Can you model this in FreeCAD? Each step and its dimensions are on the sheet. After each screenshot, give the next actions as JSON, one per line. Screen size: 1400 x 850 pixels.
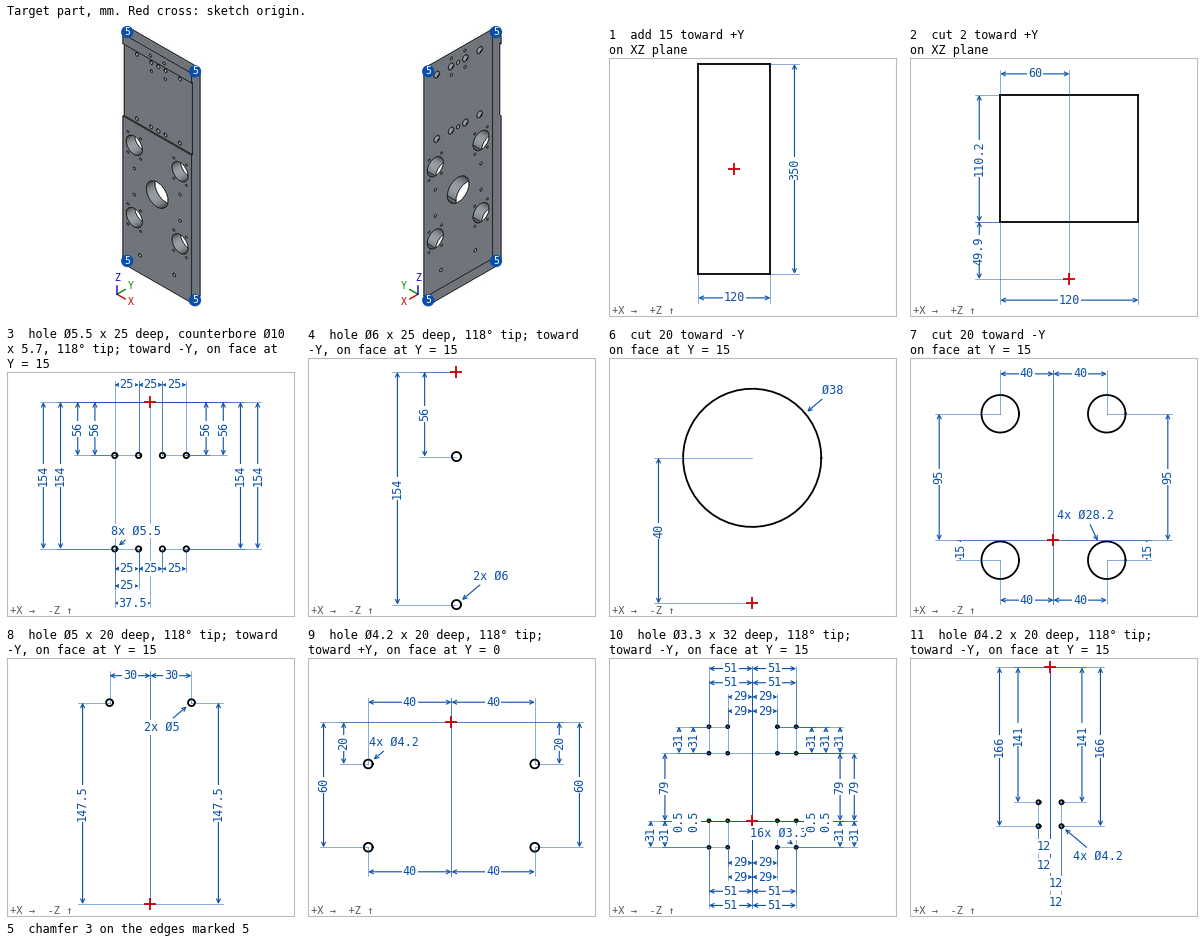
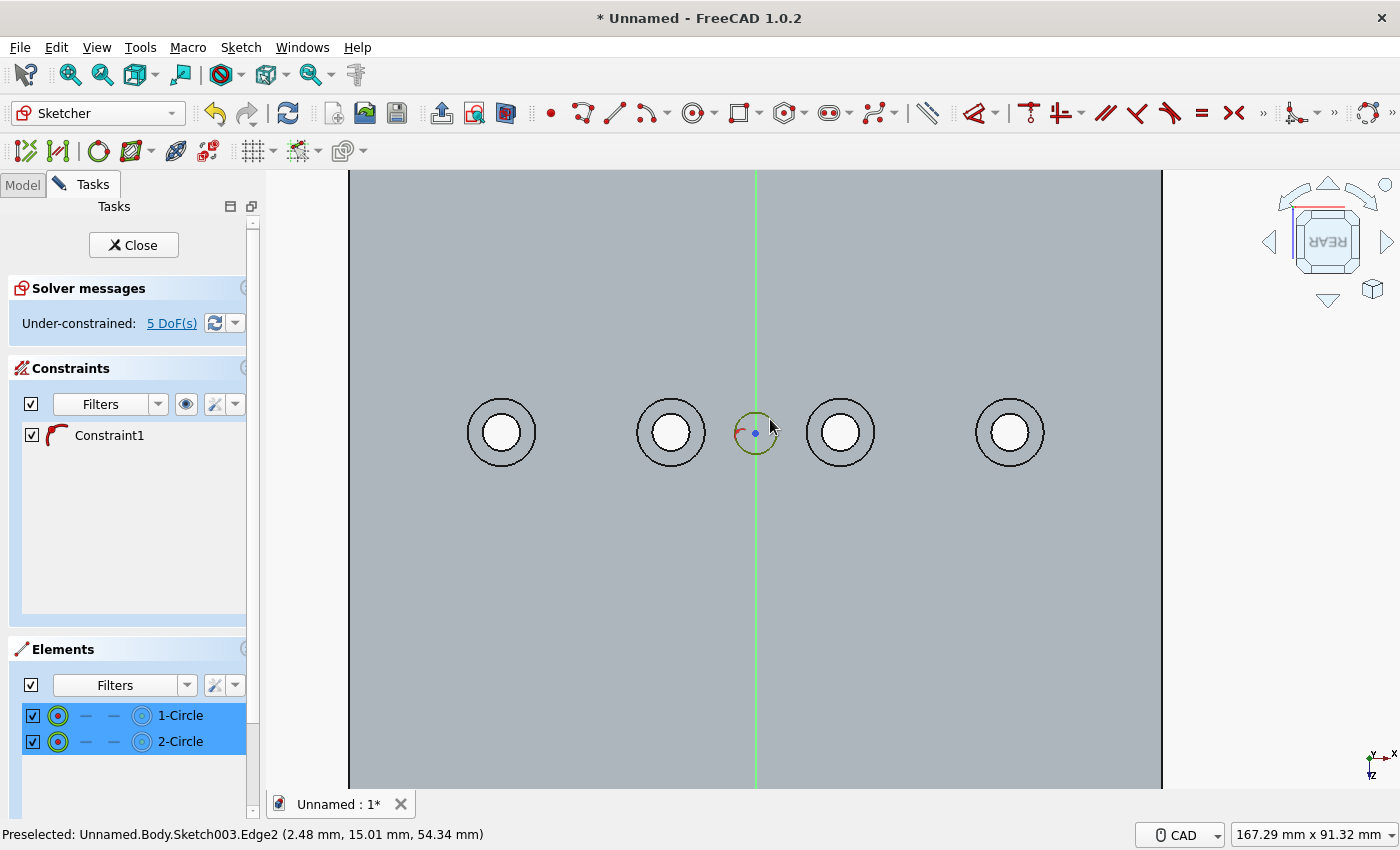
{"action": "key", "text": "e"}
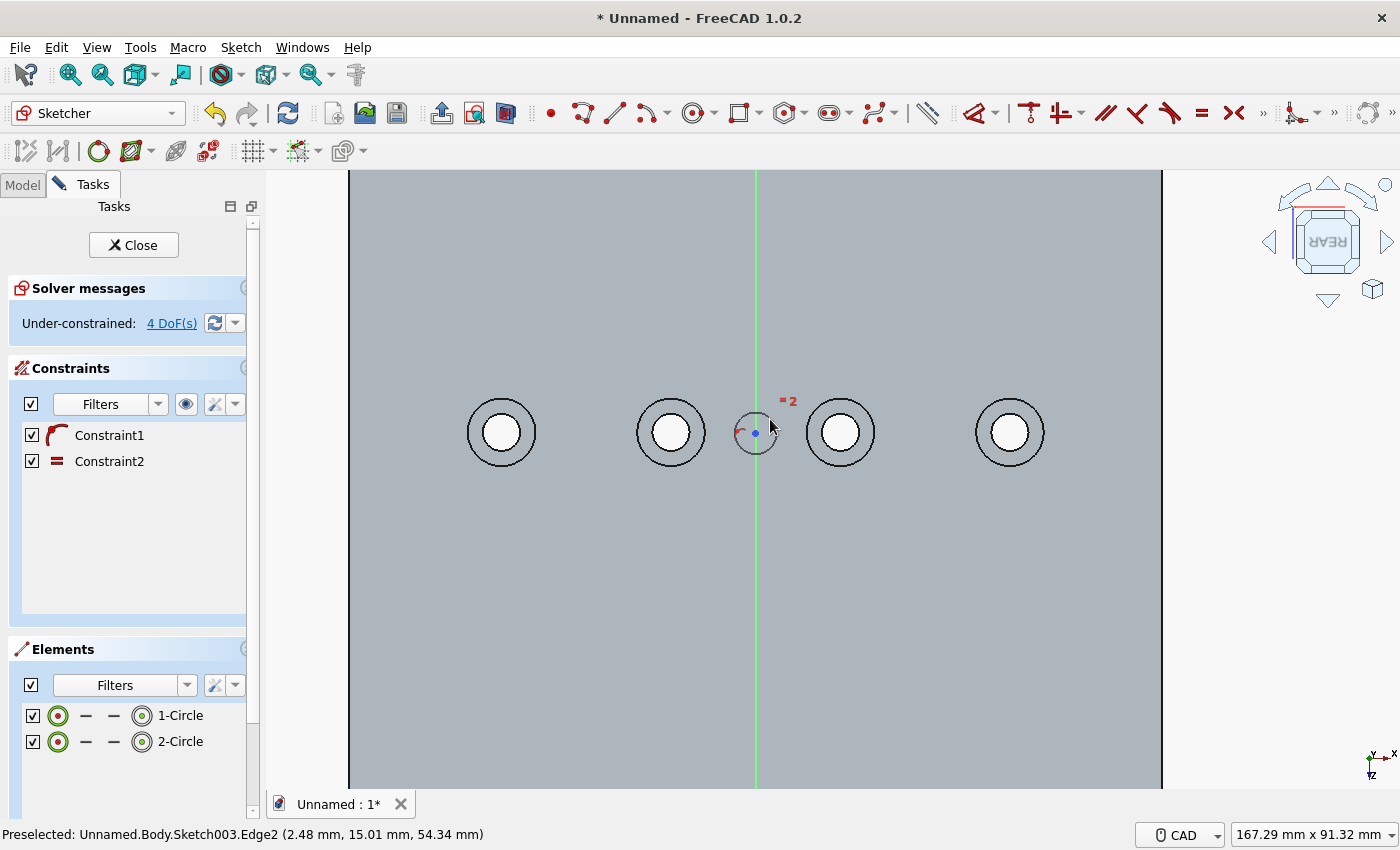
{"action": "scroll", "coordinate": [770, 418], "scroll_direction": "down", "scroll_amount": 5}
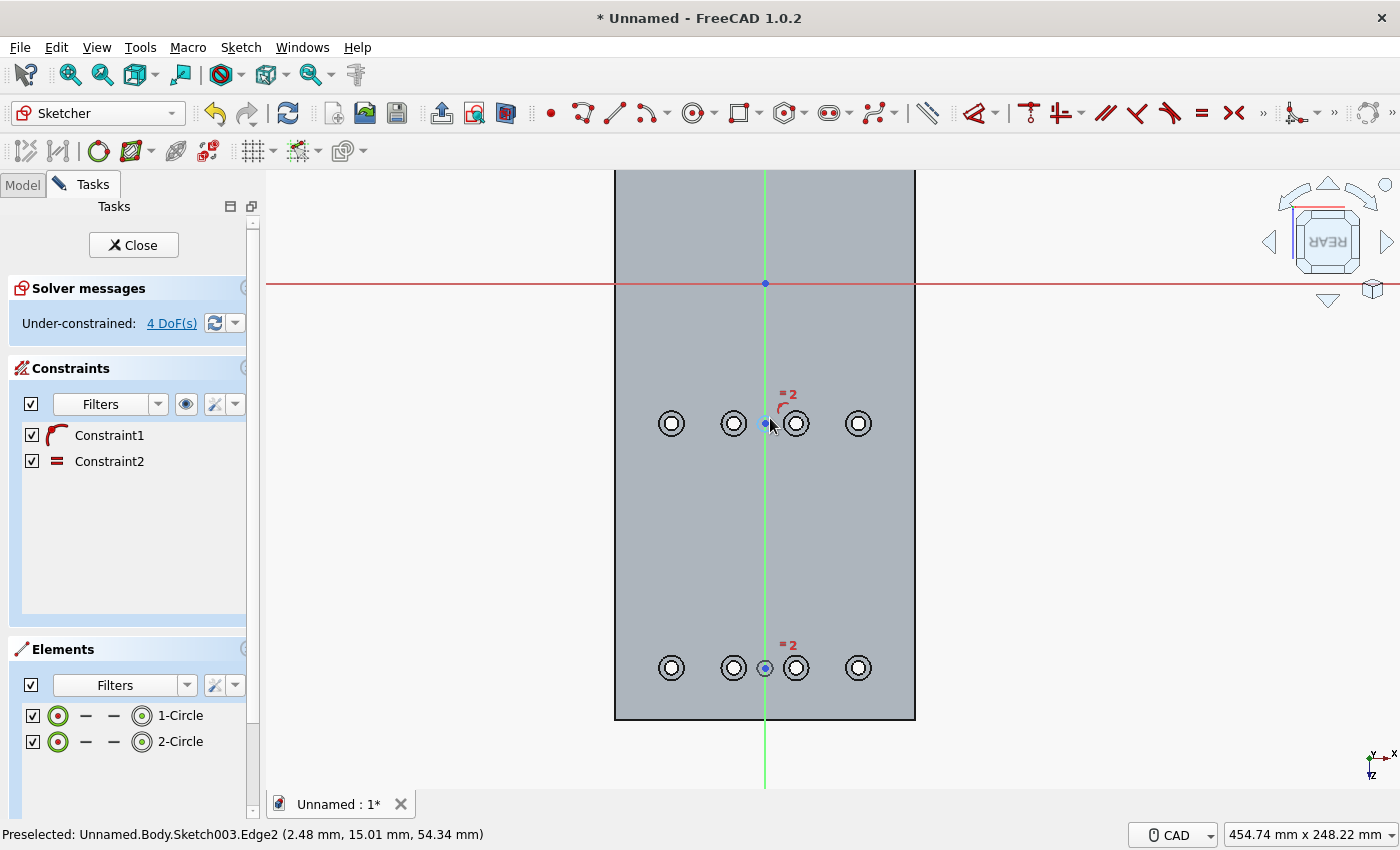
{"action": "left_click", "coordinate": [765, 668]}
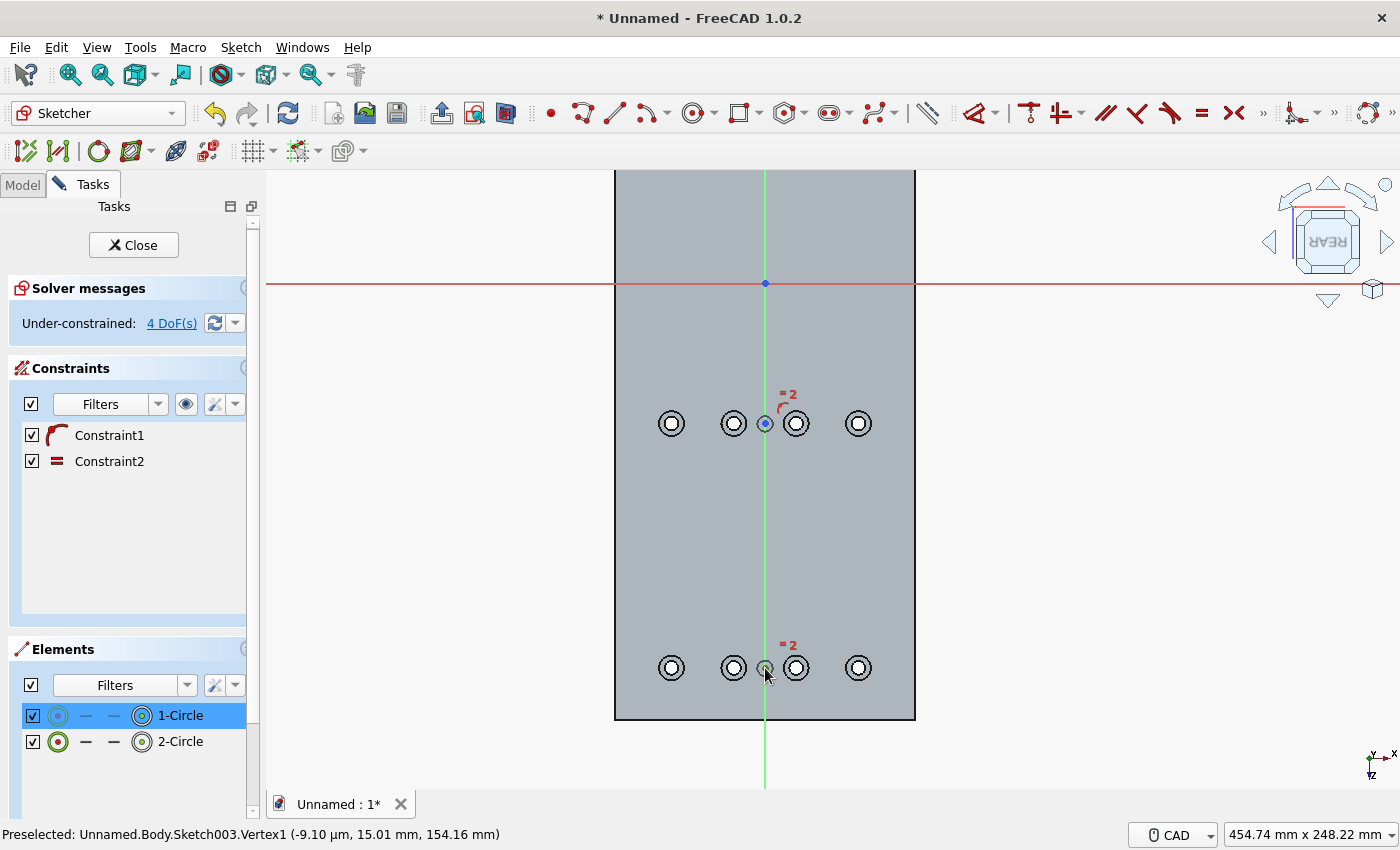
{"action": "left_click", "coordinate": [765, 721]}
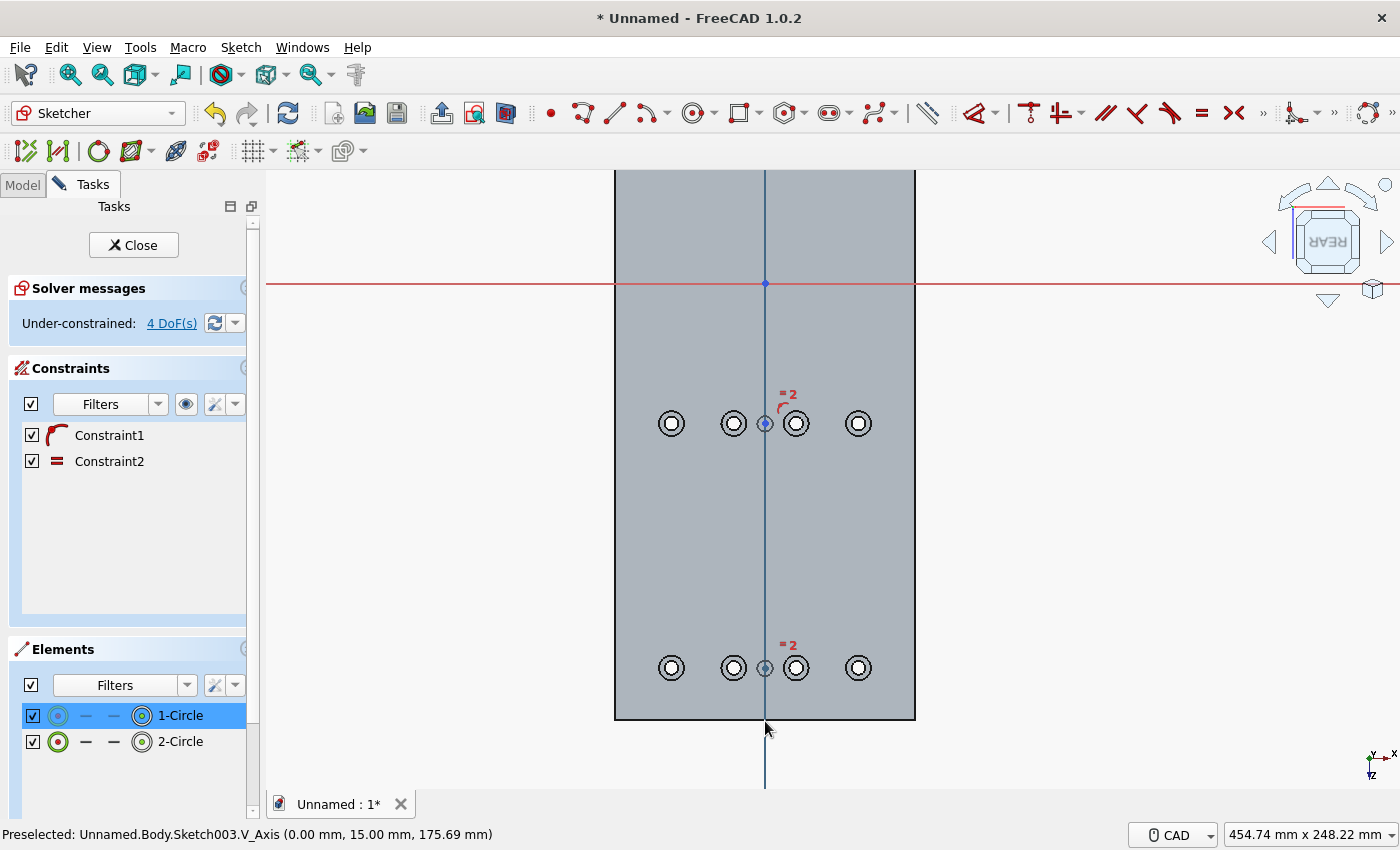
{"action": "left_click", "coordinate": [1030, 114]}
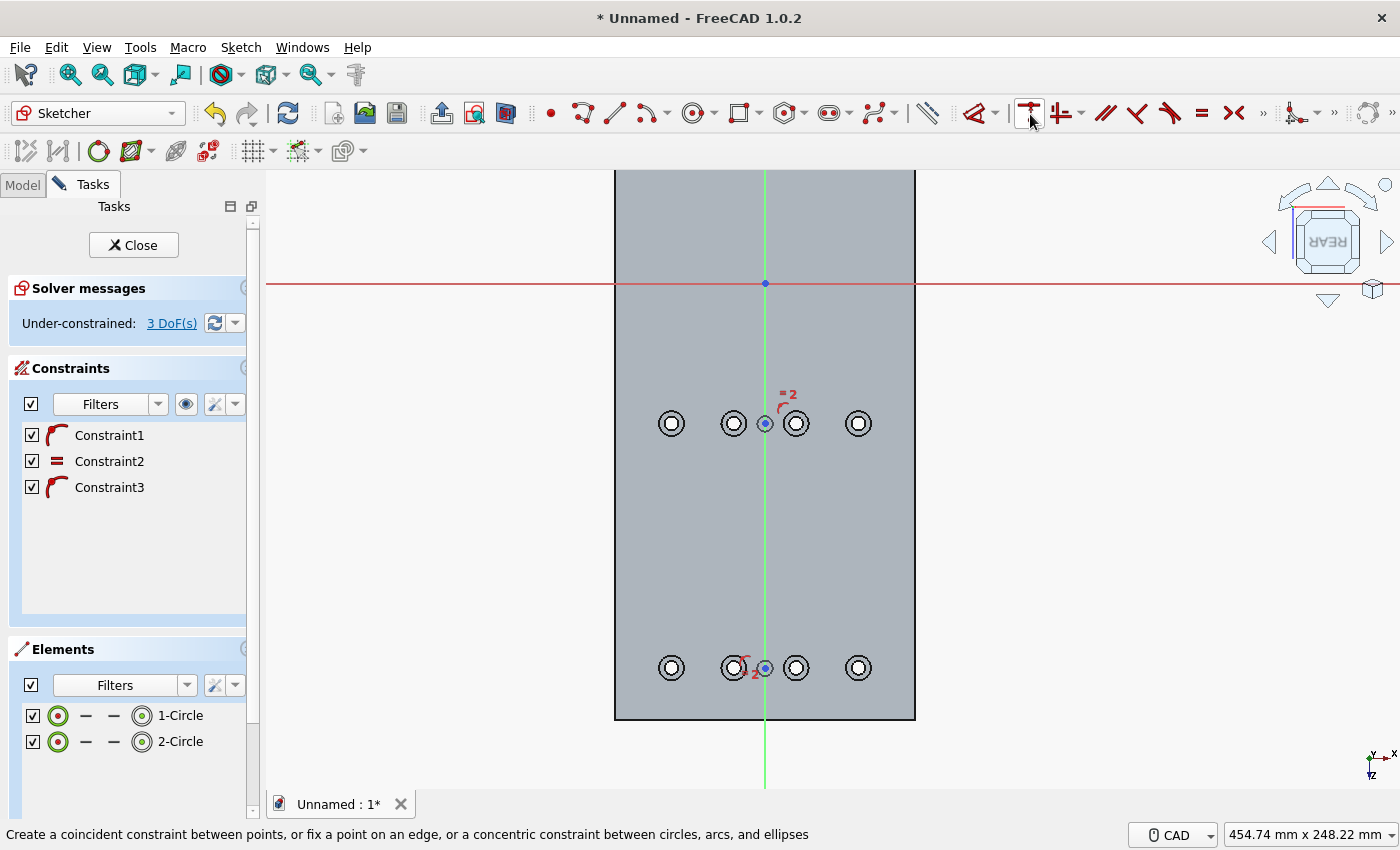
{"action": "left_click", "coordinate": [974, 114]}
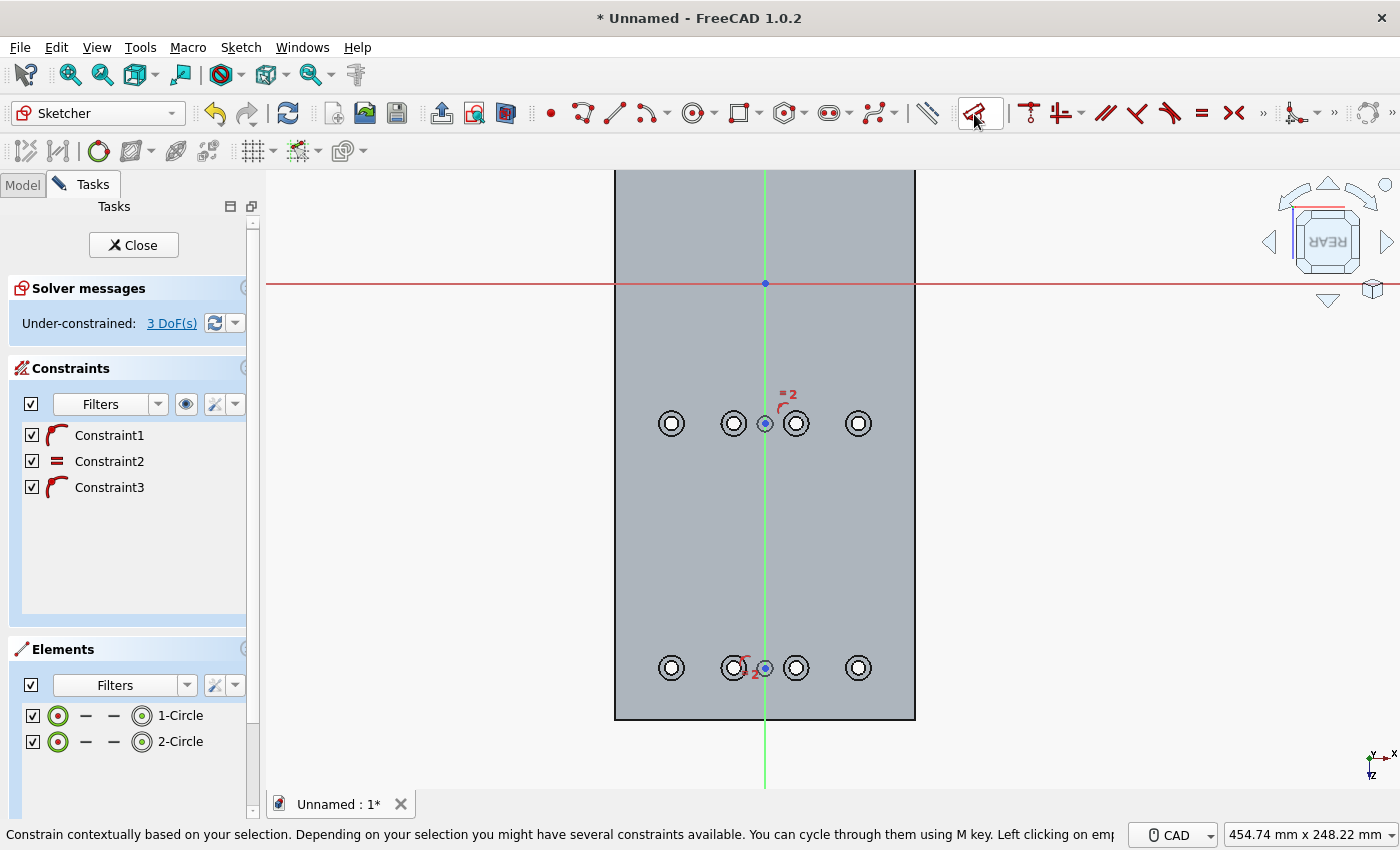
{"action": "scroll", "coordinate": [765, 661], "scroll_direction": "up", "scroll_amount": 5}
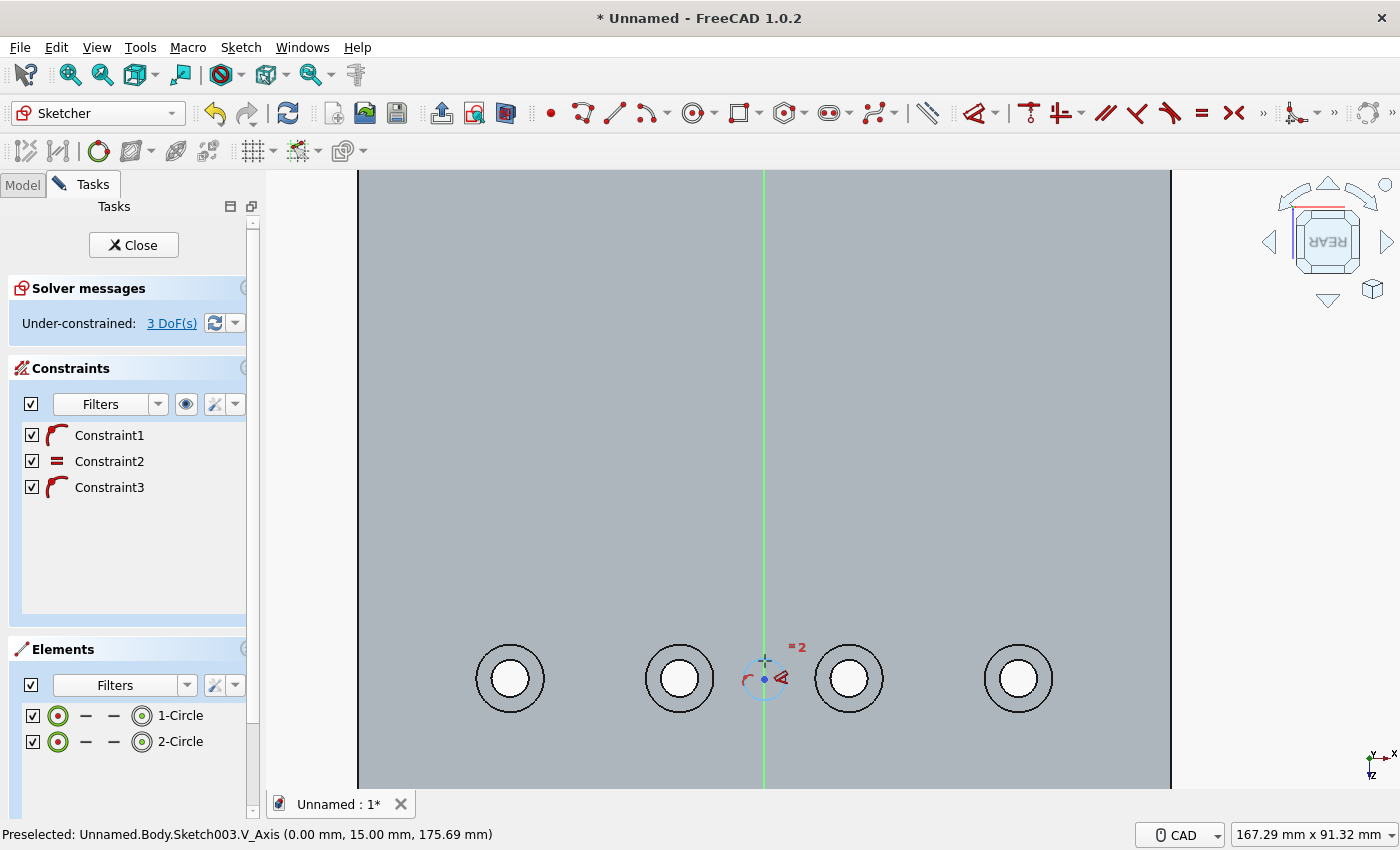
{"action": "left_click", "coordinate": [765, 659]}
{"action": "left_click", "coordinate": [791, 634]}